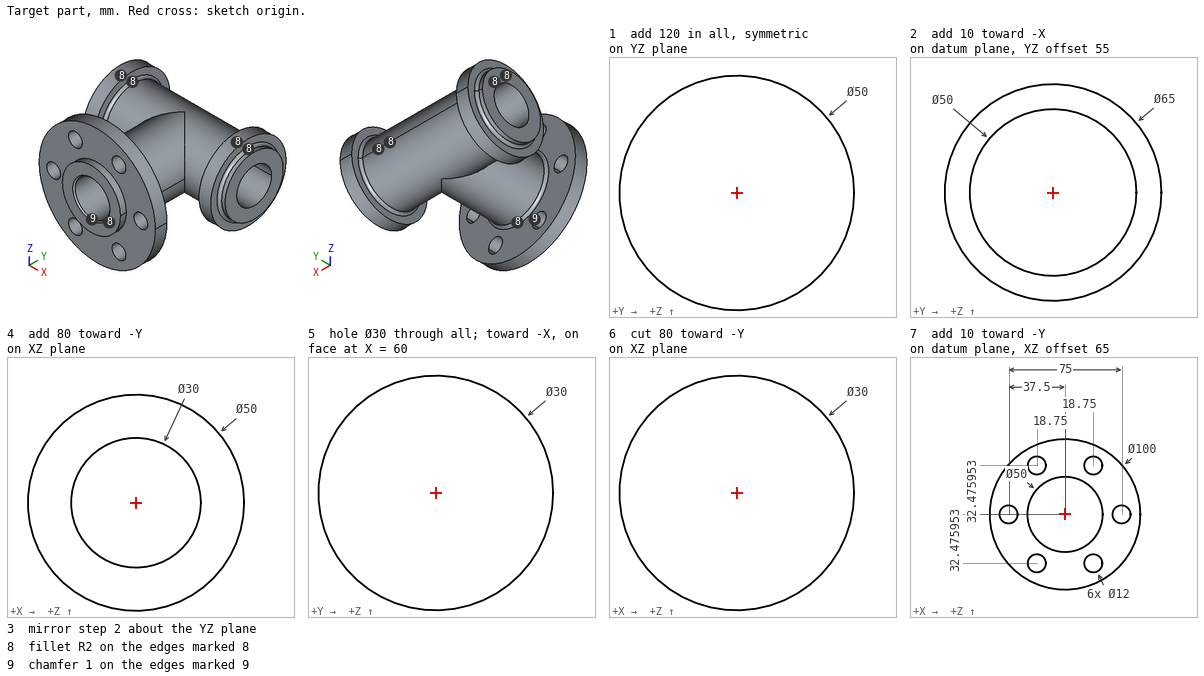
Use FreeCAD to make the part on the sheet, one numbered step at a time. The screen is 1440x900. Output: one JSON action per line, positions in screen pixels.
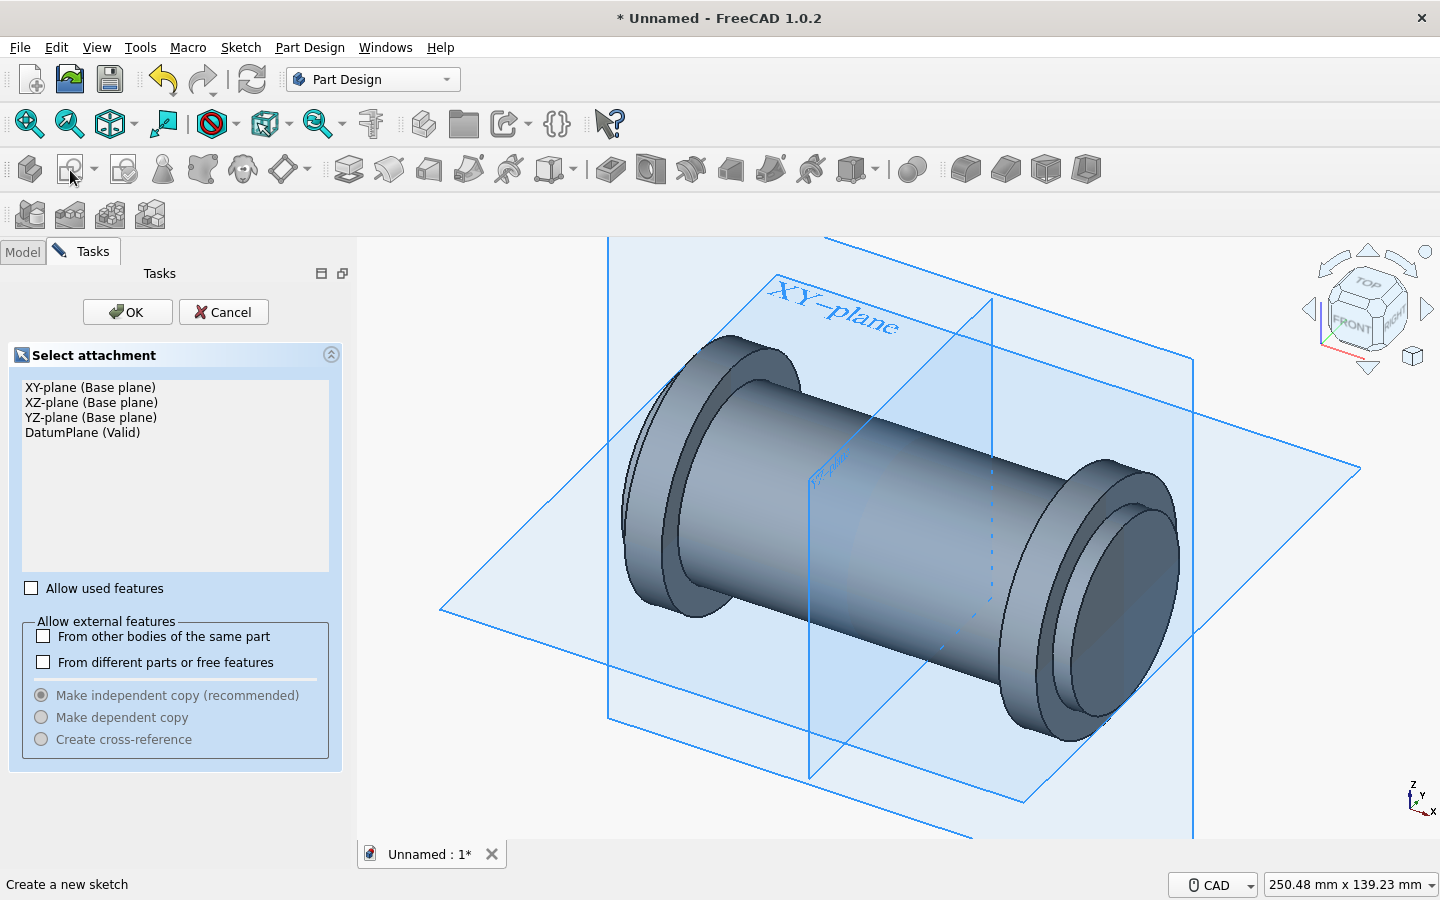
{"action": "left_click", "coordinate": [82, 402]}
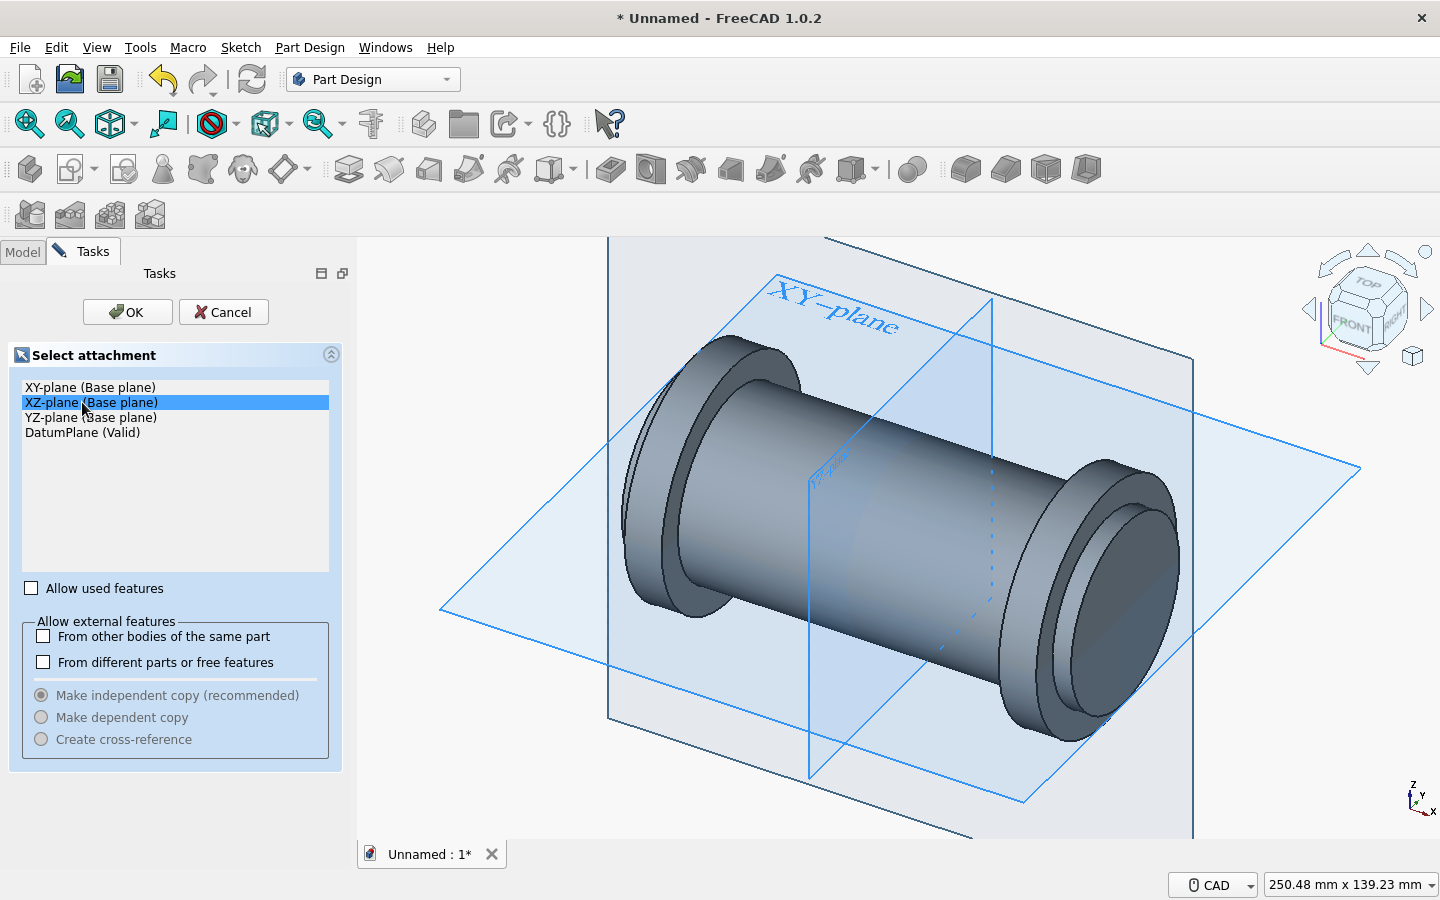
{"action": "left_click", "coordinate": [128, 312]}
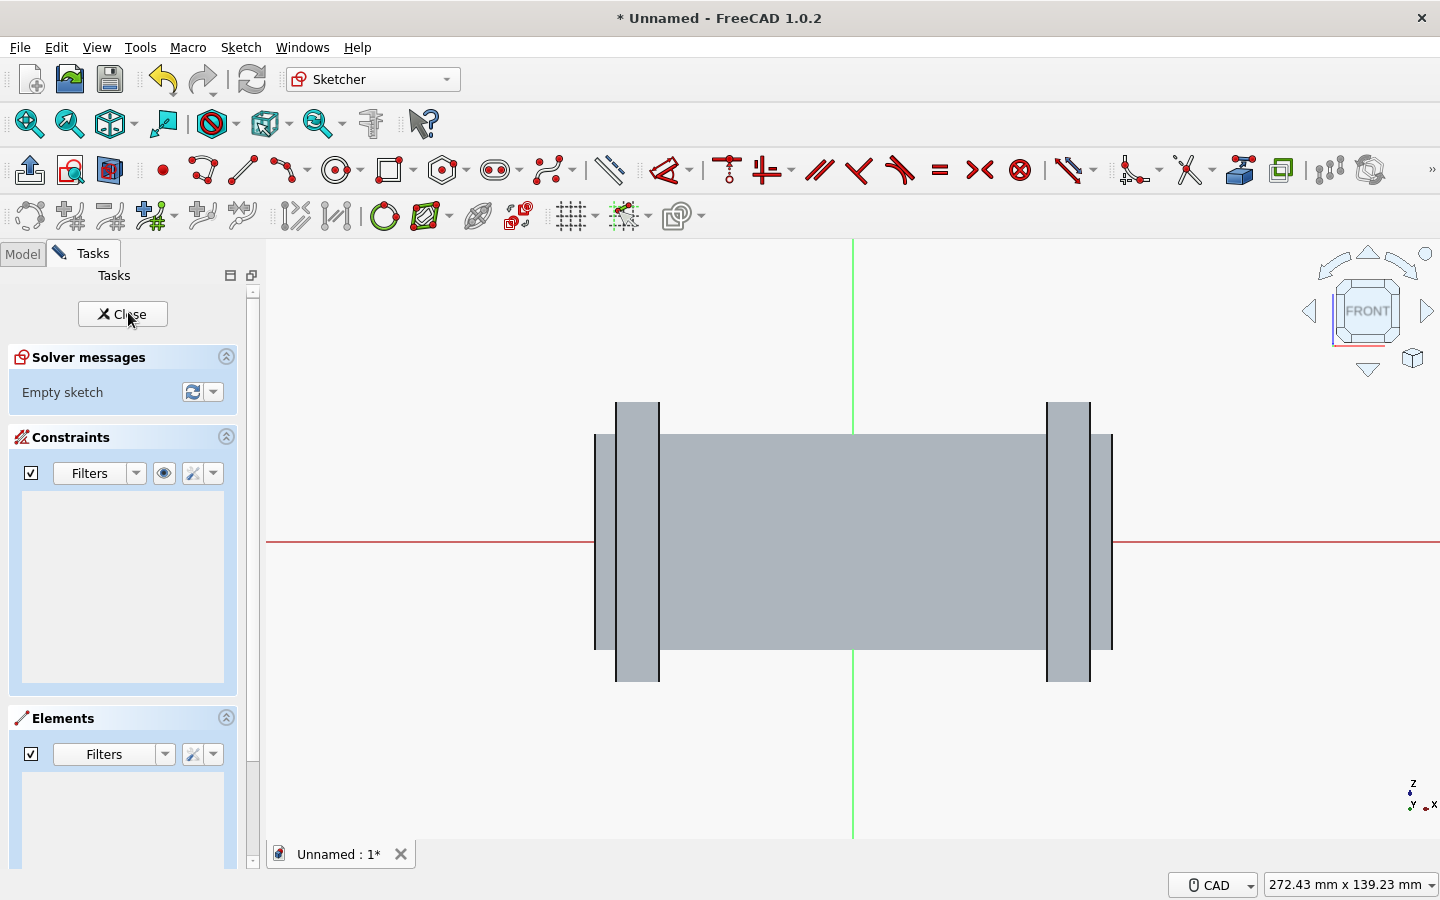
{"action": "key", "text": "q s"}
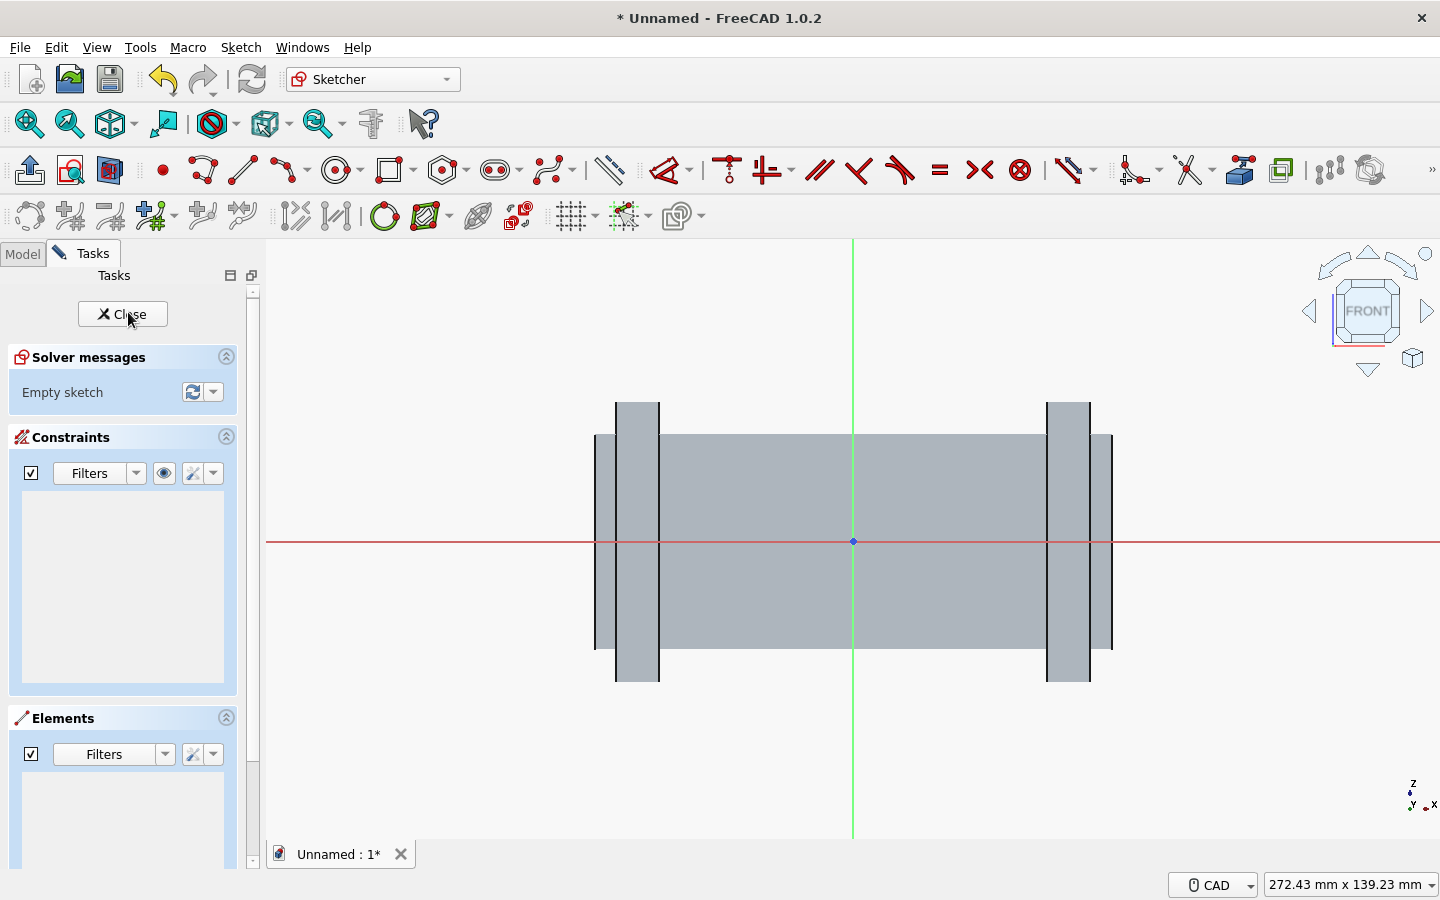
{"action": "scroll", "coordinate": [937, 546], "scroll_direction": "up", "scroll_amount": 3}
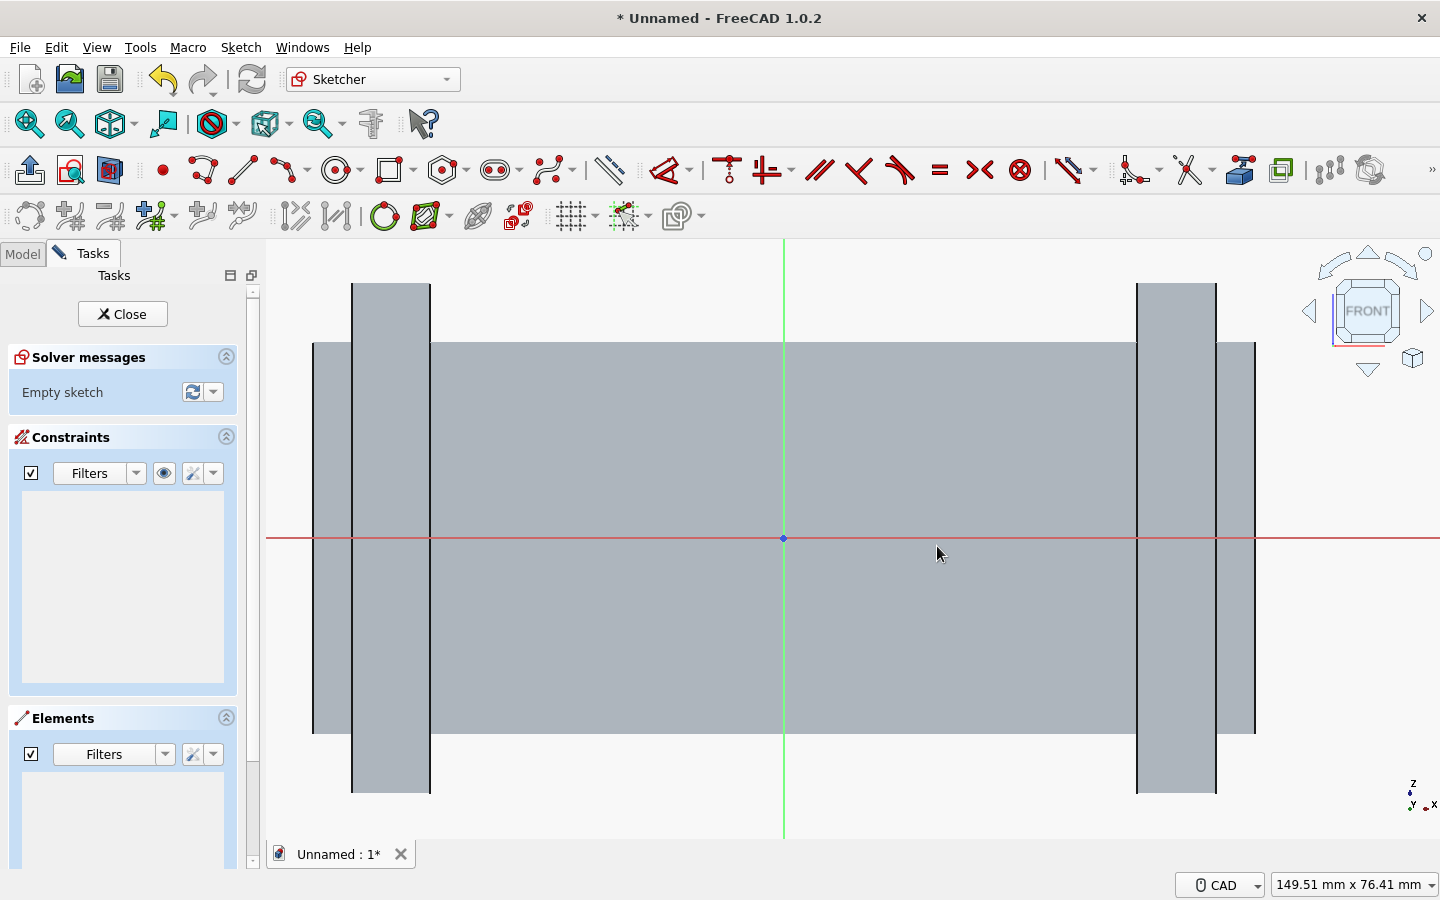
{"action": "key", "text": "g c"}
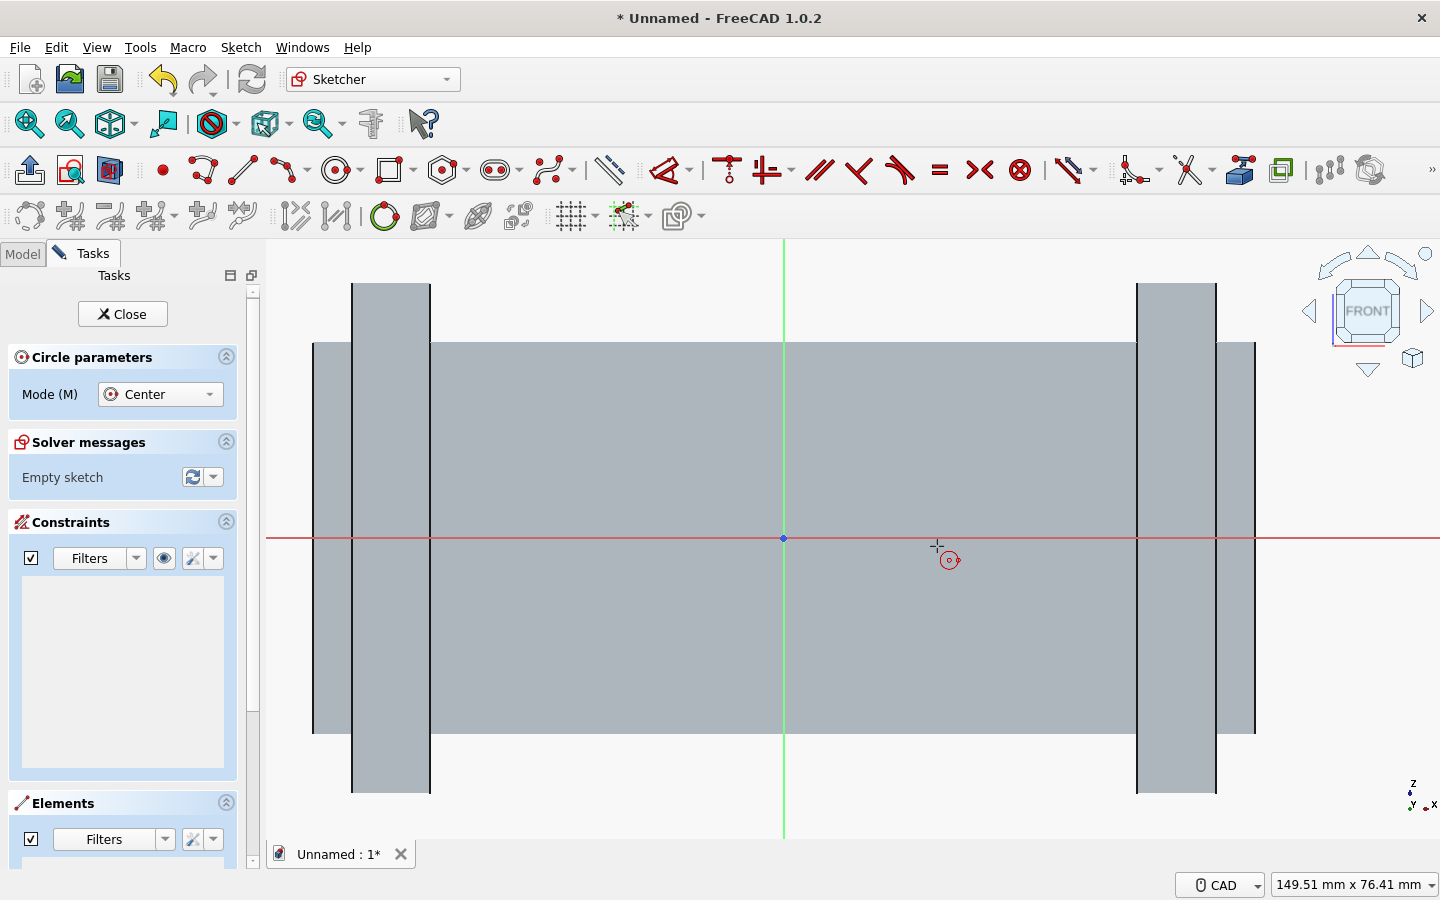
{"action": "left_click", "coordinate": [784, 538]}
{"action": "left_click", "coordinate": [923, 399]}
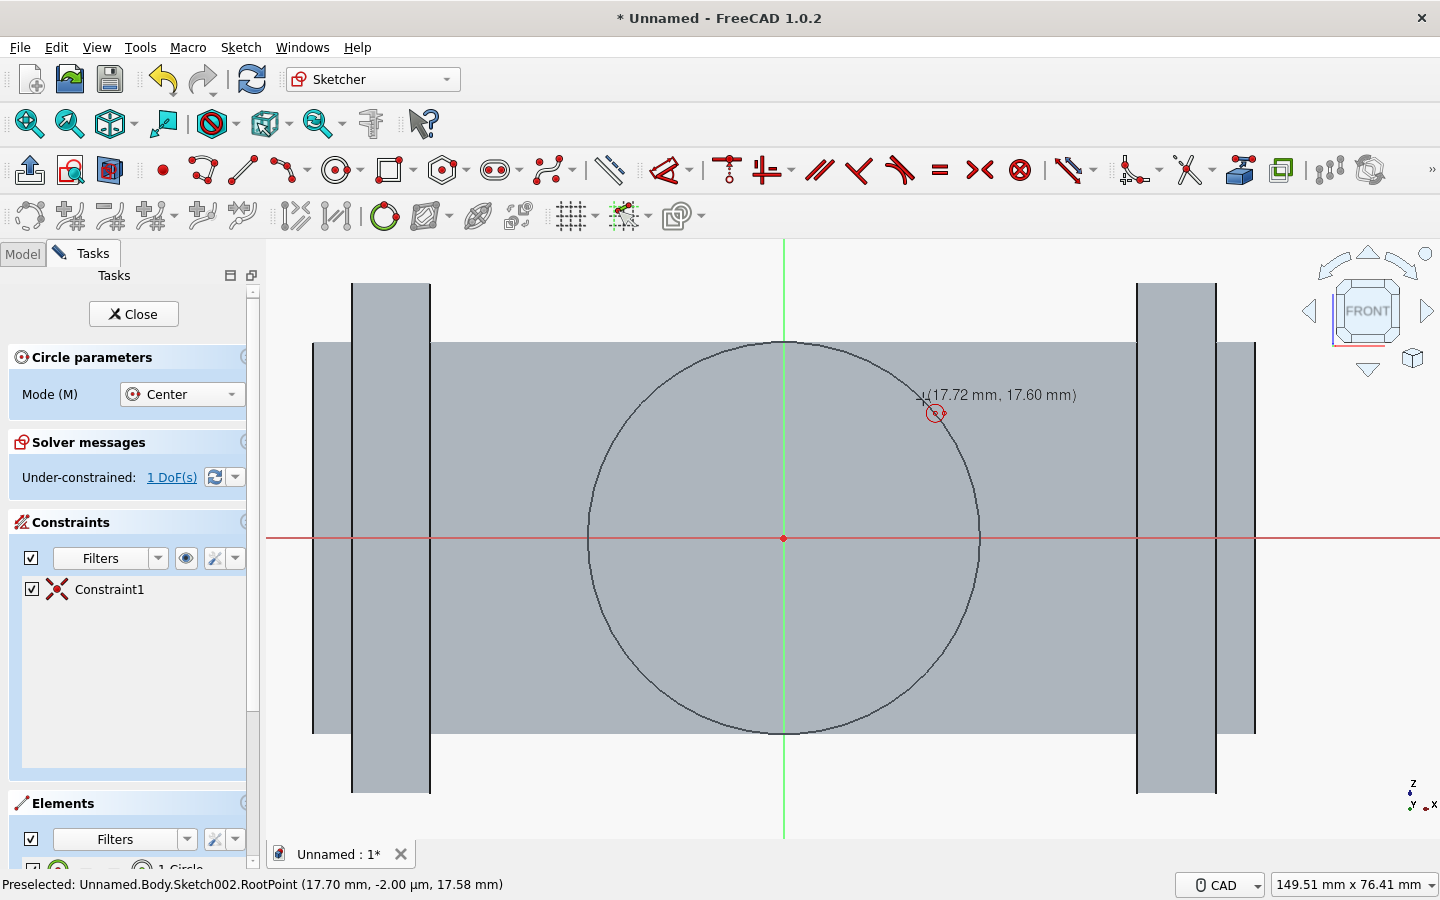
{"action": "left_click", "coordinate": [784, 538]}
{"action": "left_click", "coordinate": [867, 455]}
{"action": "key", "text": "Escape"}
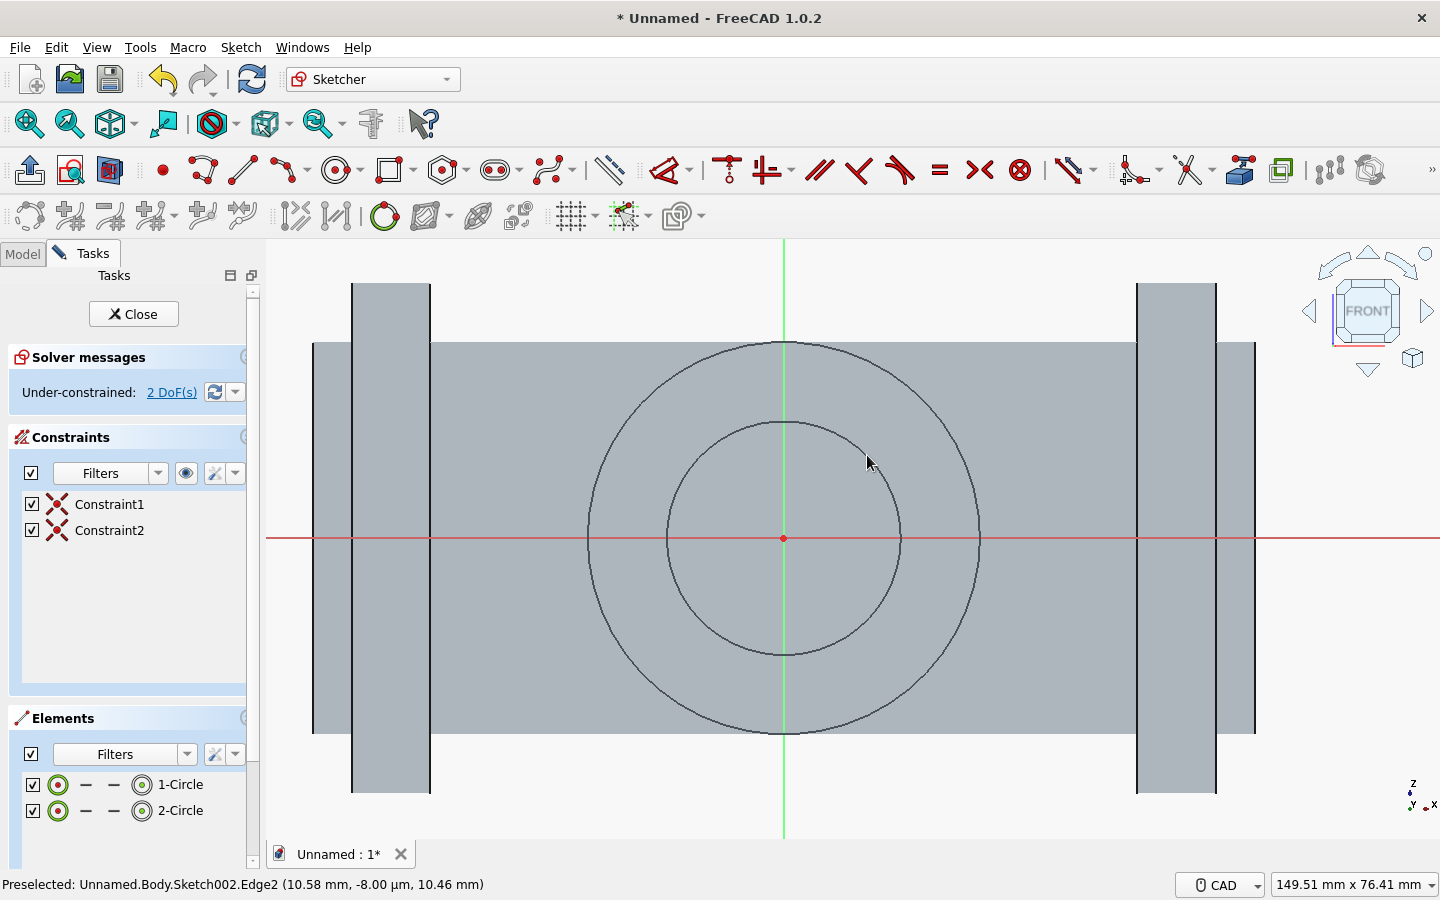
{"action": "left_click", "coordinate": [922, 399]}